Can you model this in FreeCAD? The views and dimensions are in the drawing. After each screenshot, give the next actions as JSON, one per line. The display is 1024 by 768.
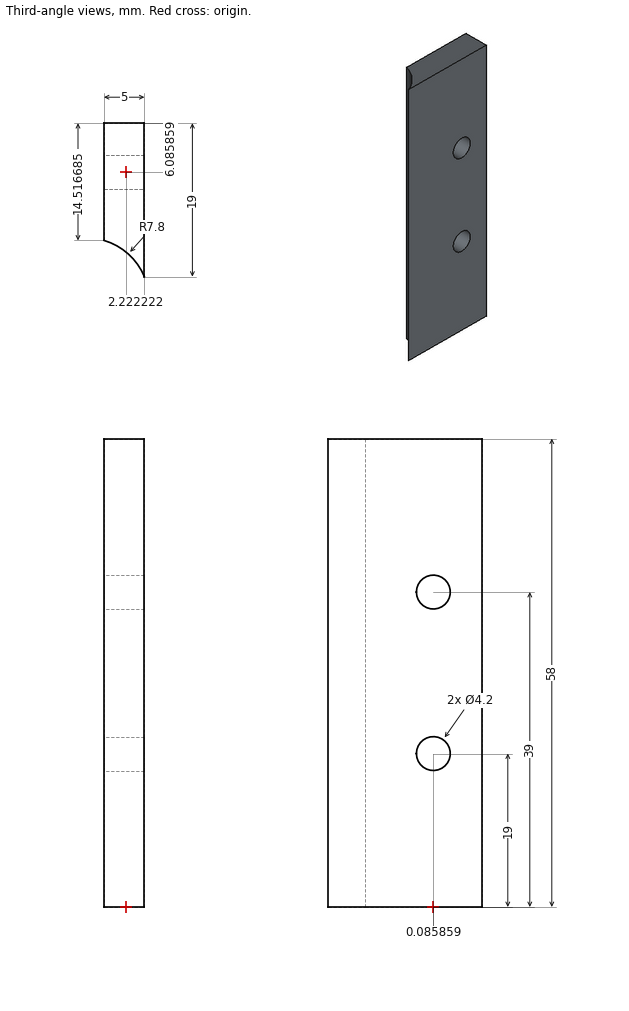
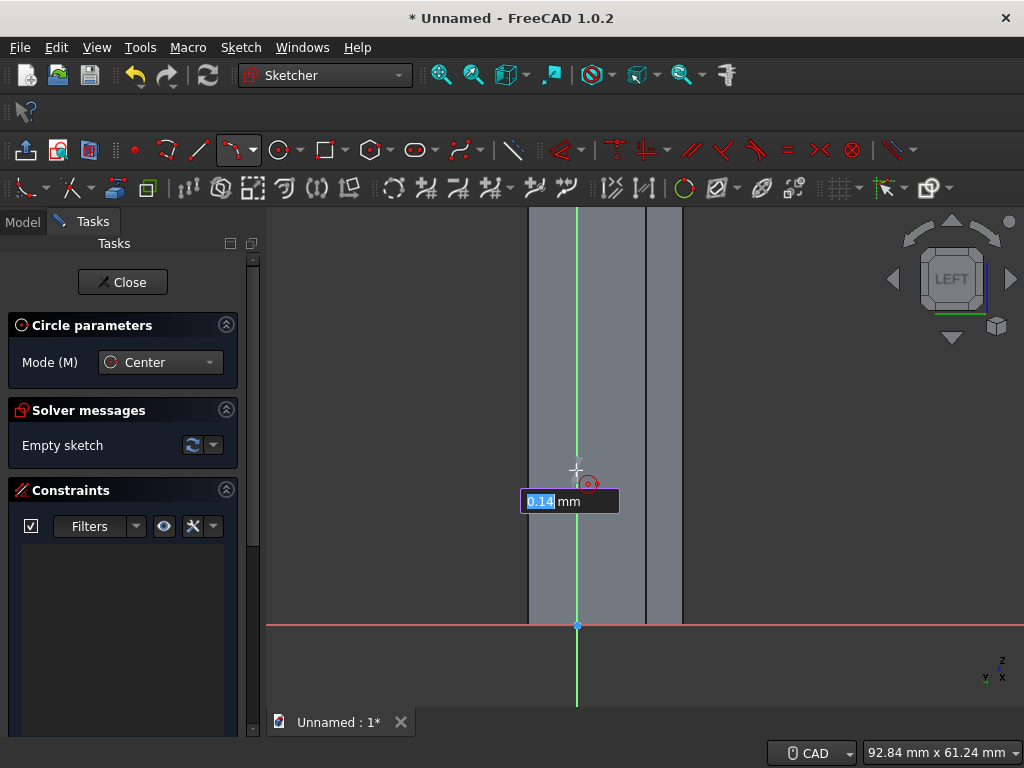
{"action": "scroll", "coordinate": [589, 458], "scroll_direction": "up", "scroll_amount": 2}
{"action": "mouse_move", "coordinate": [588, 457]}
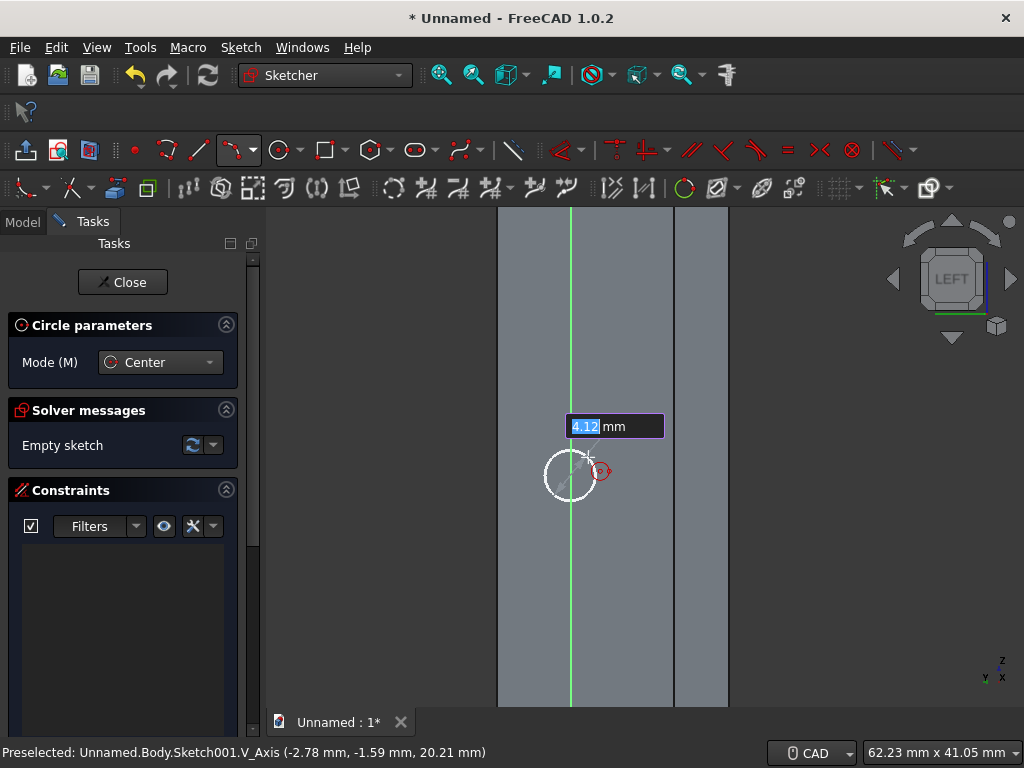
{"action": "type", "text": "4.2"}
{"action": "key", "text": "Return"}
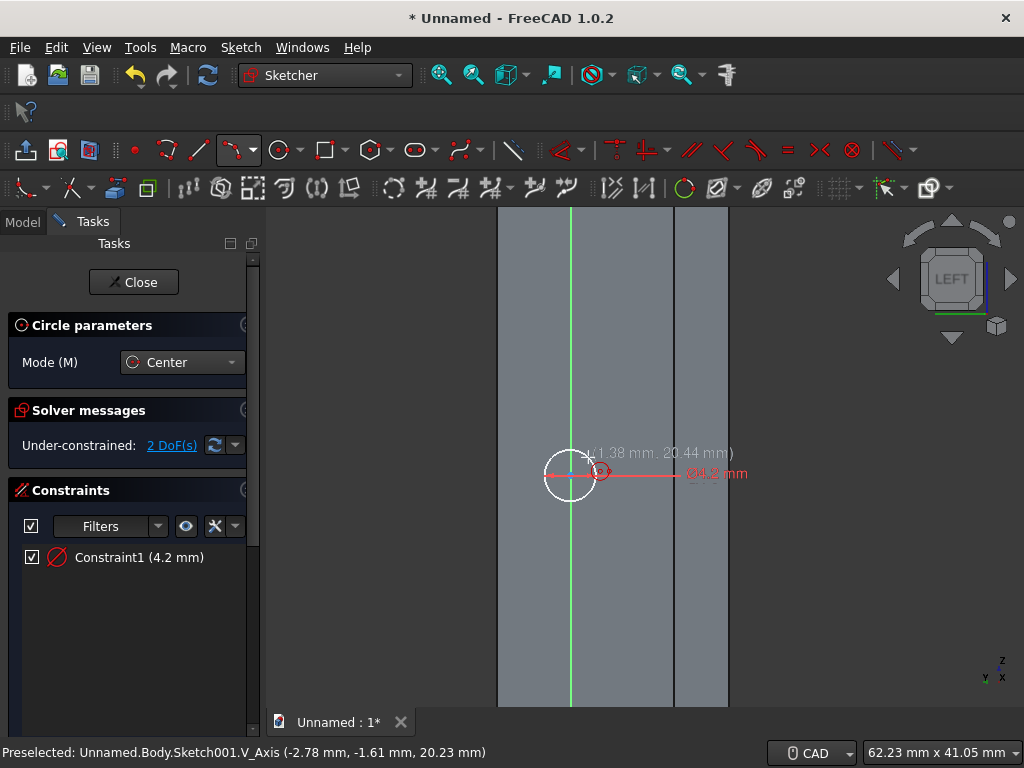
{"action": "scroll", "coordinate": [589, 458], "scroll_direction": "down", "scroll_amount": 2}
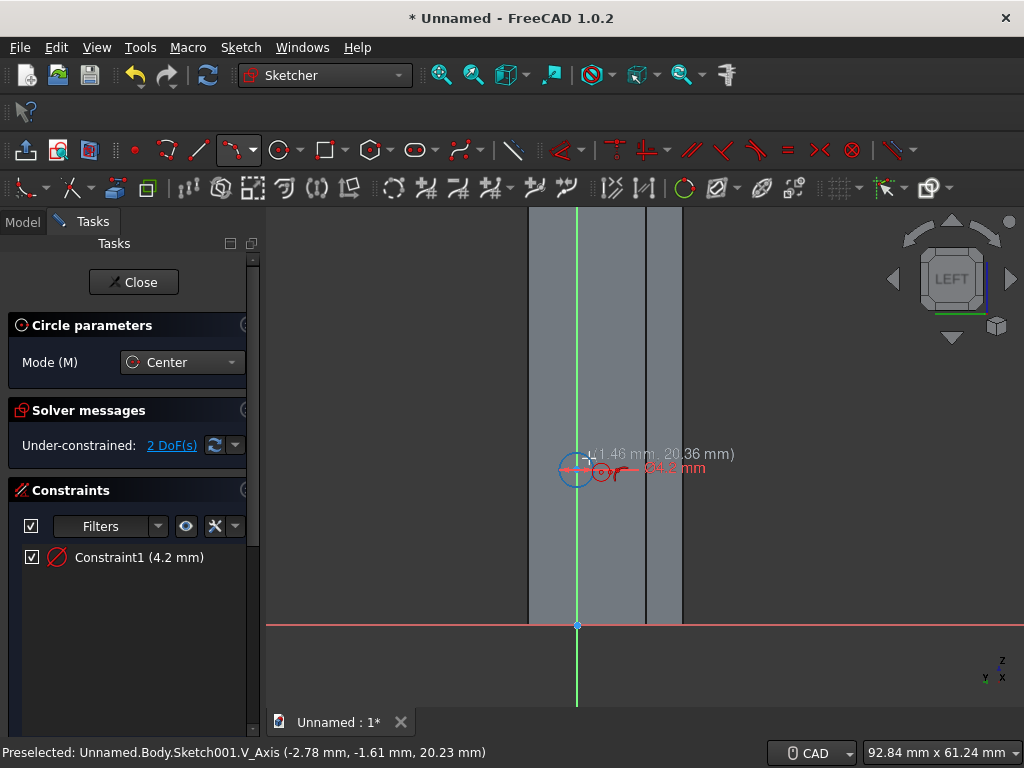
{"action": "scroll", "coordinate": [577, 307], "scroll_direction": "up", "scroll_amount": 16}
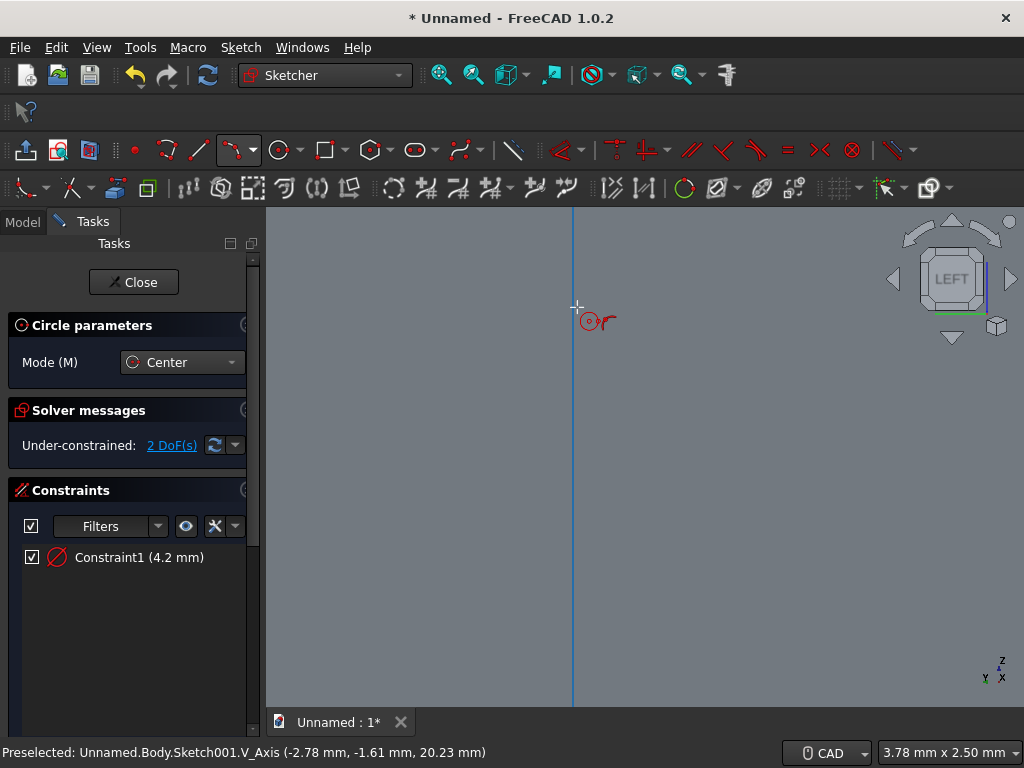
{"action": "left_click", "coordinate": [555, 294]}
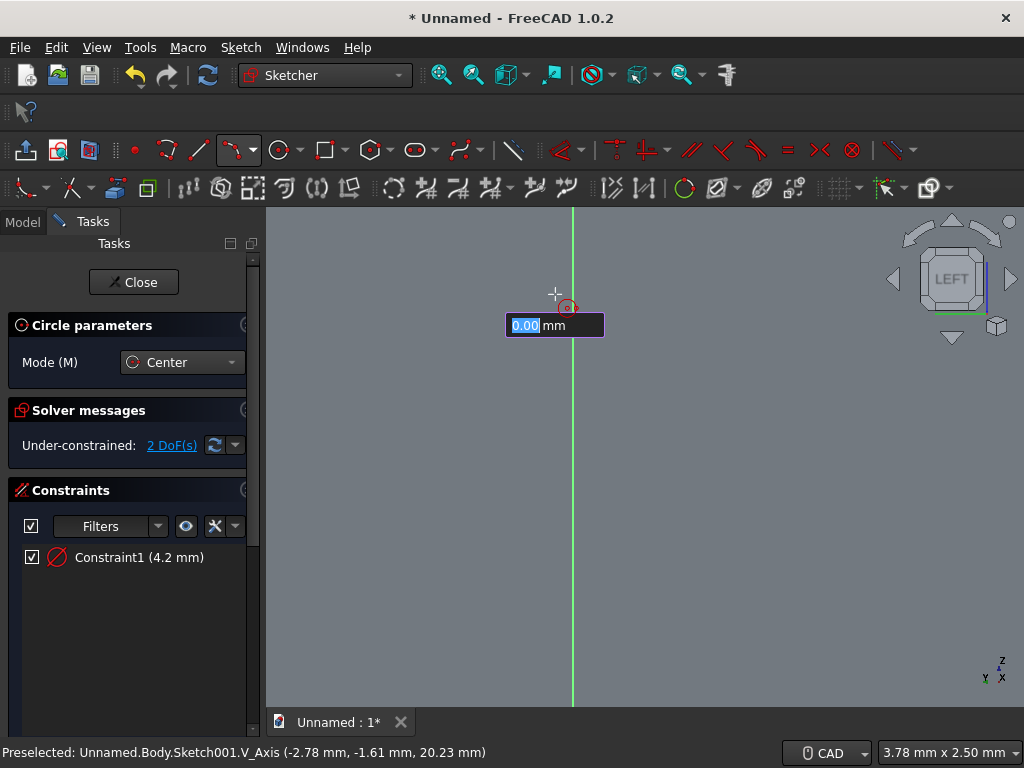
{"action": "scroll", "coordinate": [577, 307], "scroll_direction": "down", "scroll_amount": 16}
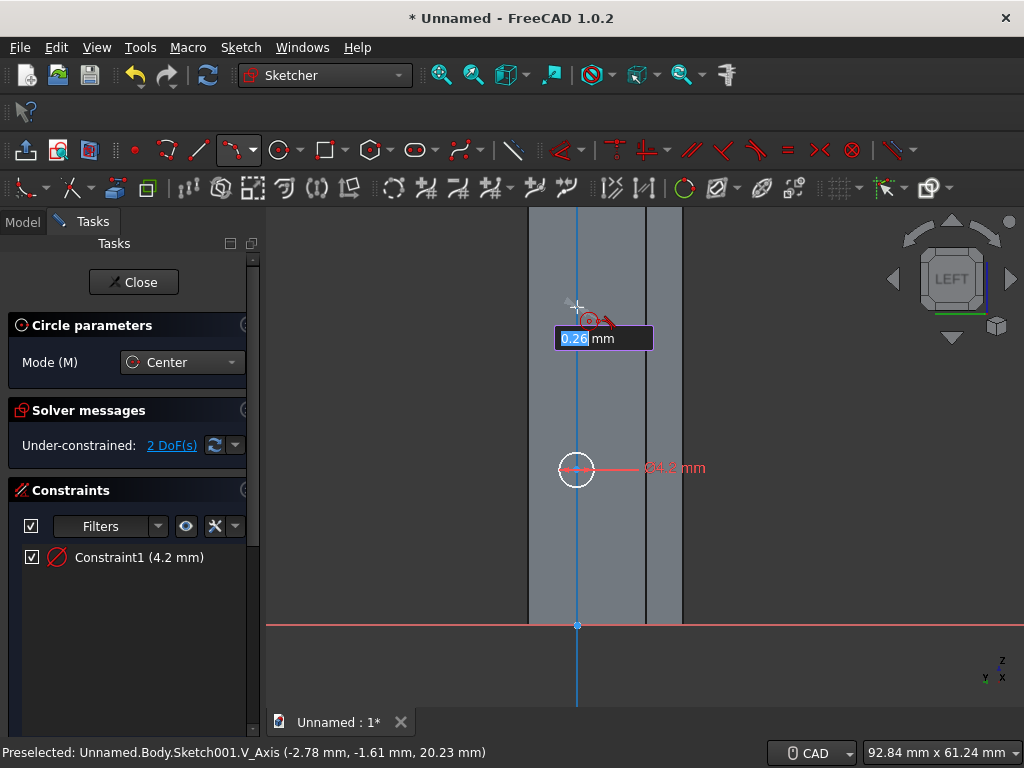
{"action": "scroll", "coordinate": [589, 295], "scroll_direction": "up", "scroll_amount": 2}
{"action": "mouse_move", "coordinate": [588, 294]}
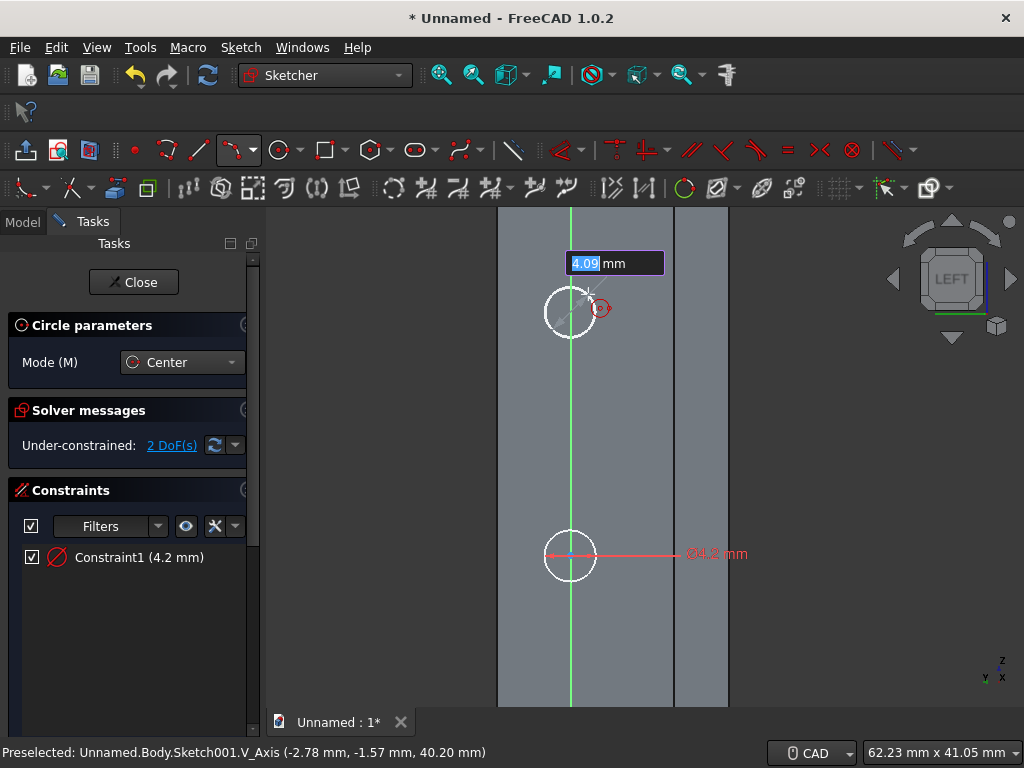
{"action": "type", "text": "4.2"}
{"action": "key", "text": "Return"}
{"action": "key", "text": "Escape"}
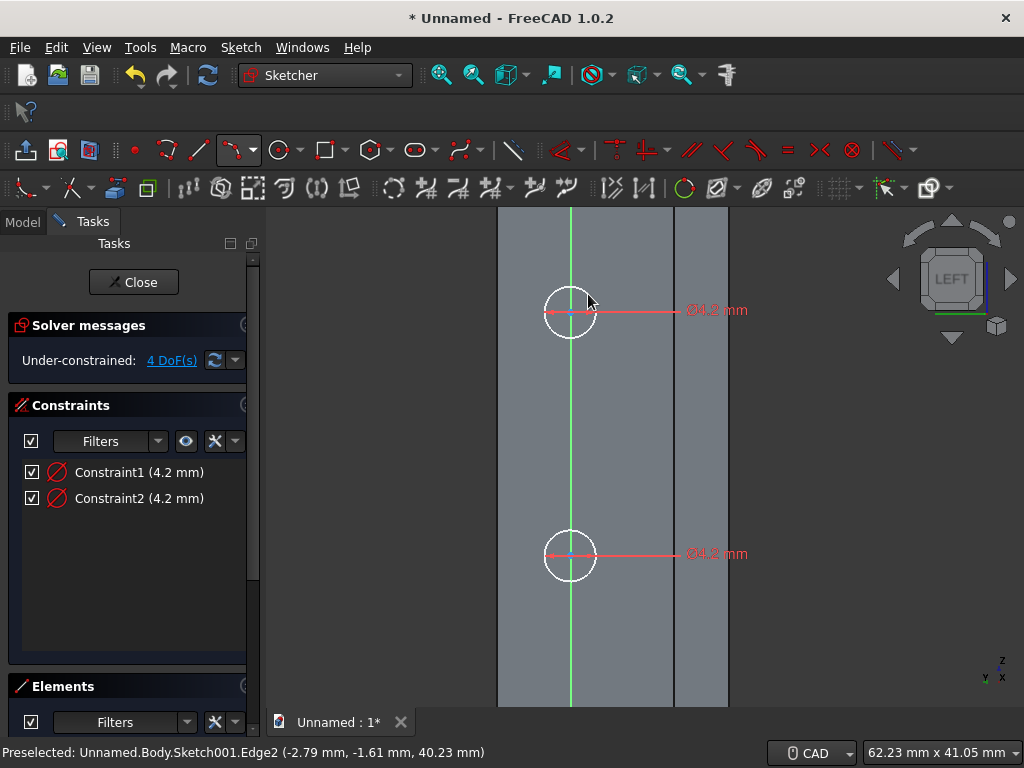
{"action": "left_click", "coordinate": [560, 150]}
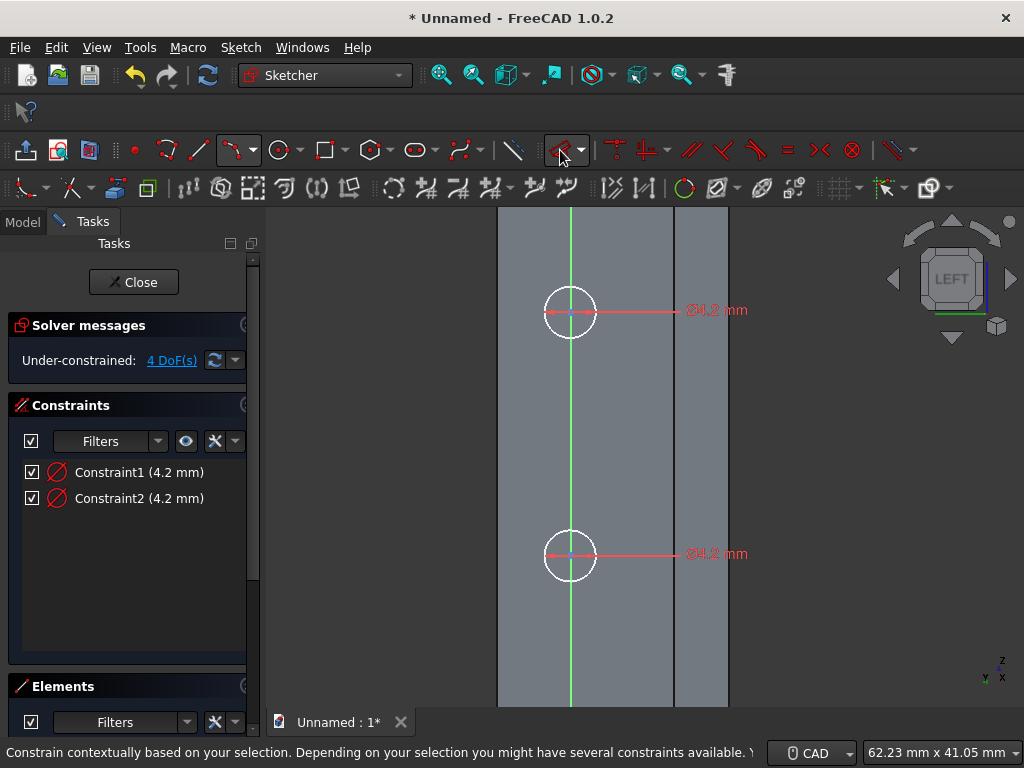
{"action": "left_click", "coordinate": [570, 556]}
{"action": "left_click", "coordinate": [605, 617]}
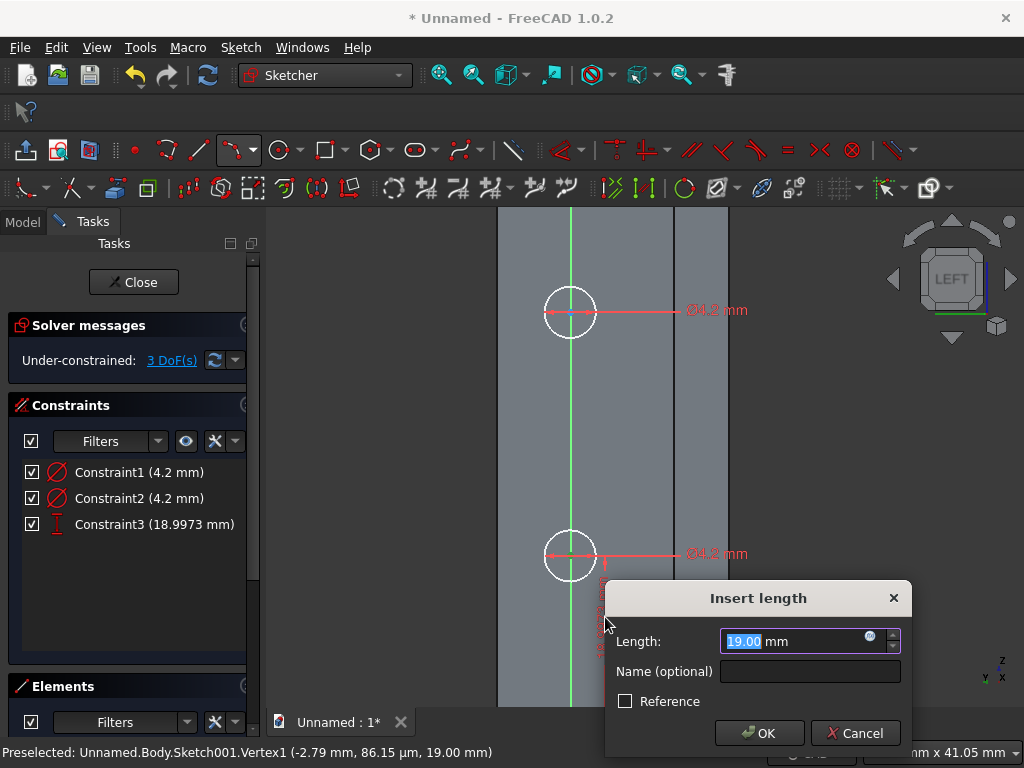
{"action": "type", "text": "19"}
{"action": "key", "text": "Return"}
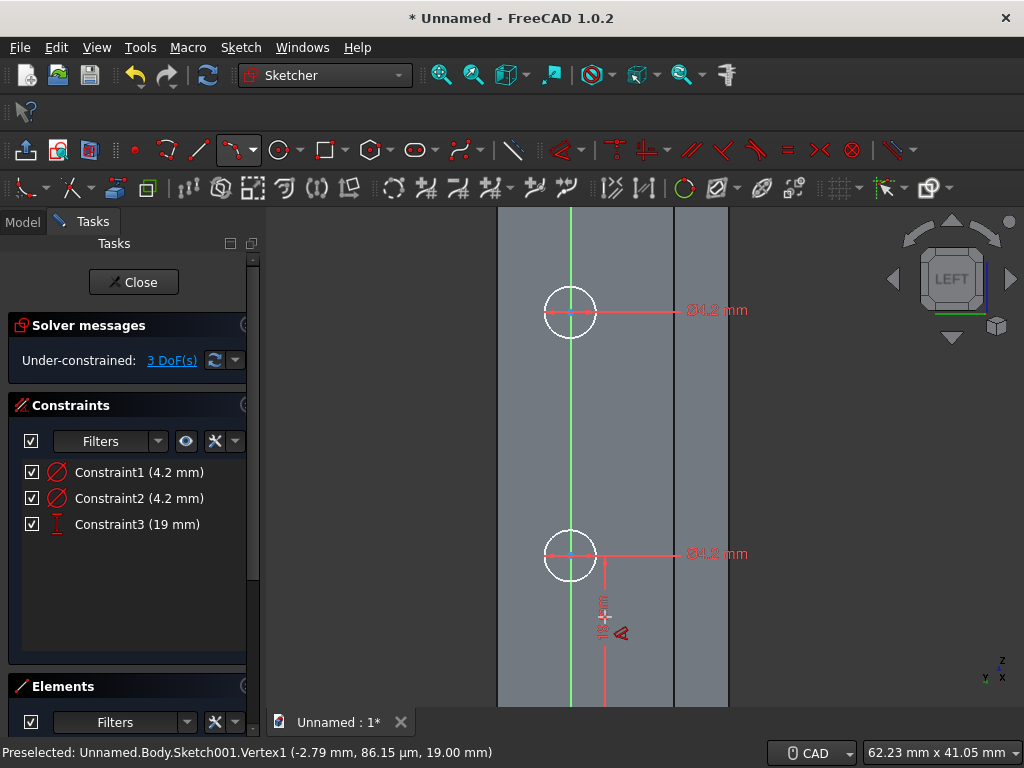
{"action": "left_click", "coordinate": [570, 312]}
{"action": "left_click", "coordinate": [605, 496]}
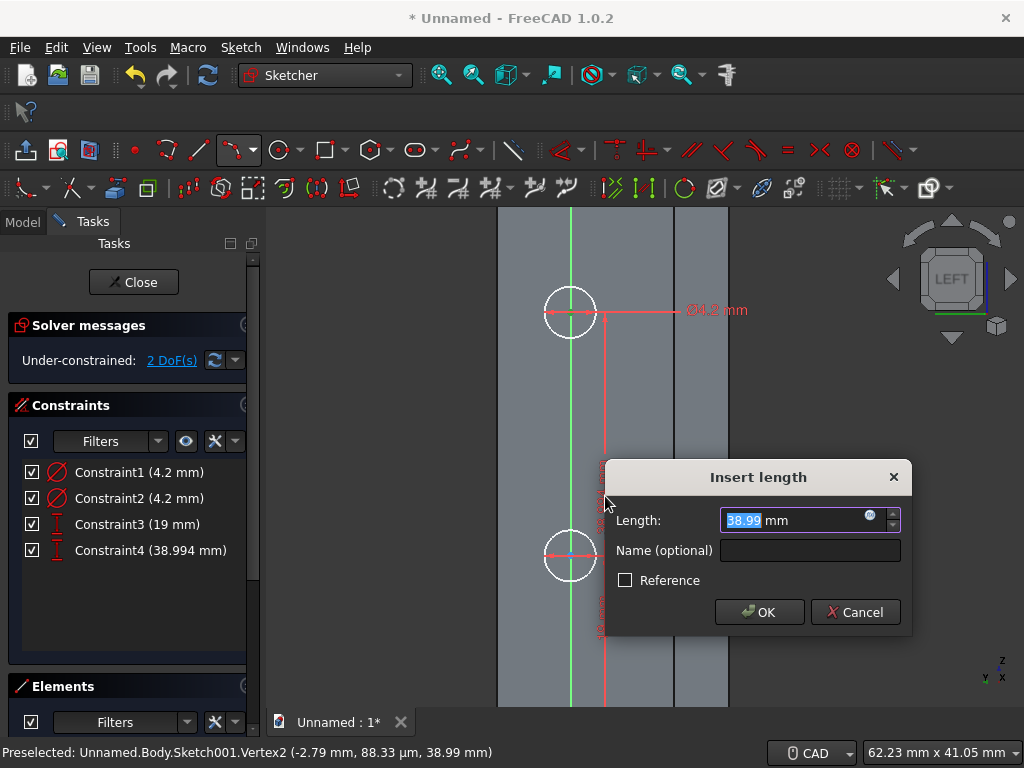
{"action": "type", "text": "39"}
{"action": "key", "text": "Return"}